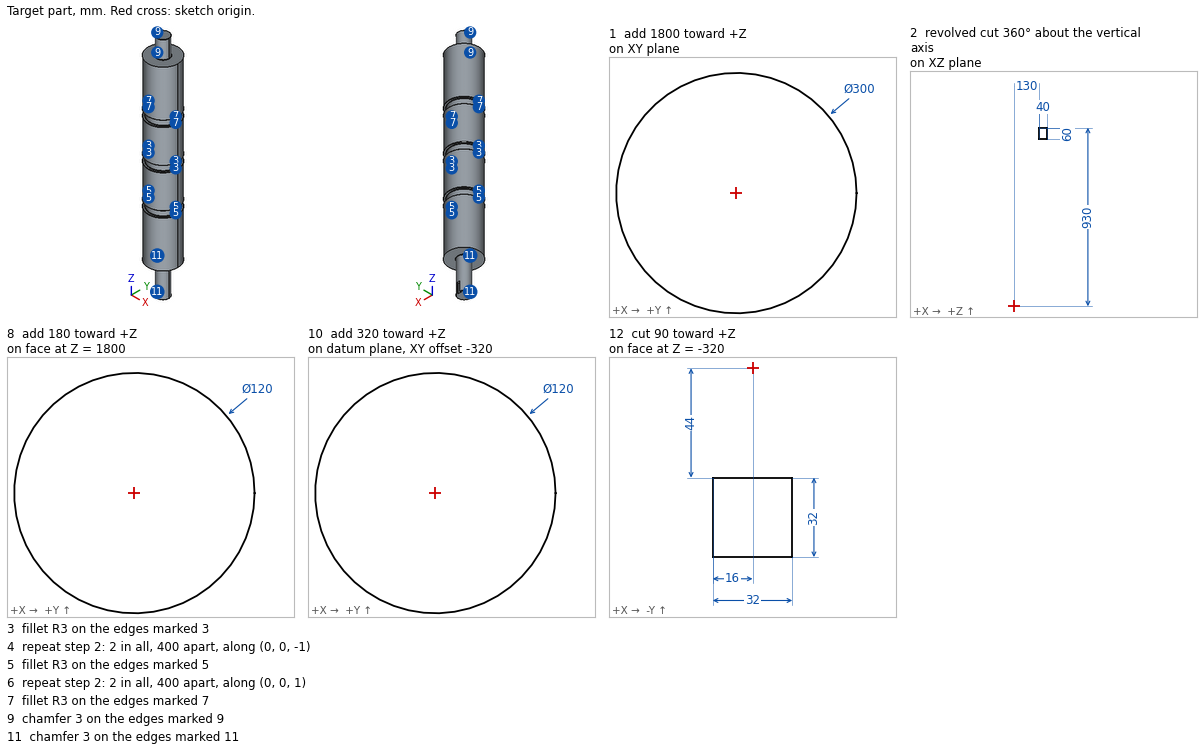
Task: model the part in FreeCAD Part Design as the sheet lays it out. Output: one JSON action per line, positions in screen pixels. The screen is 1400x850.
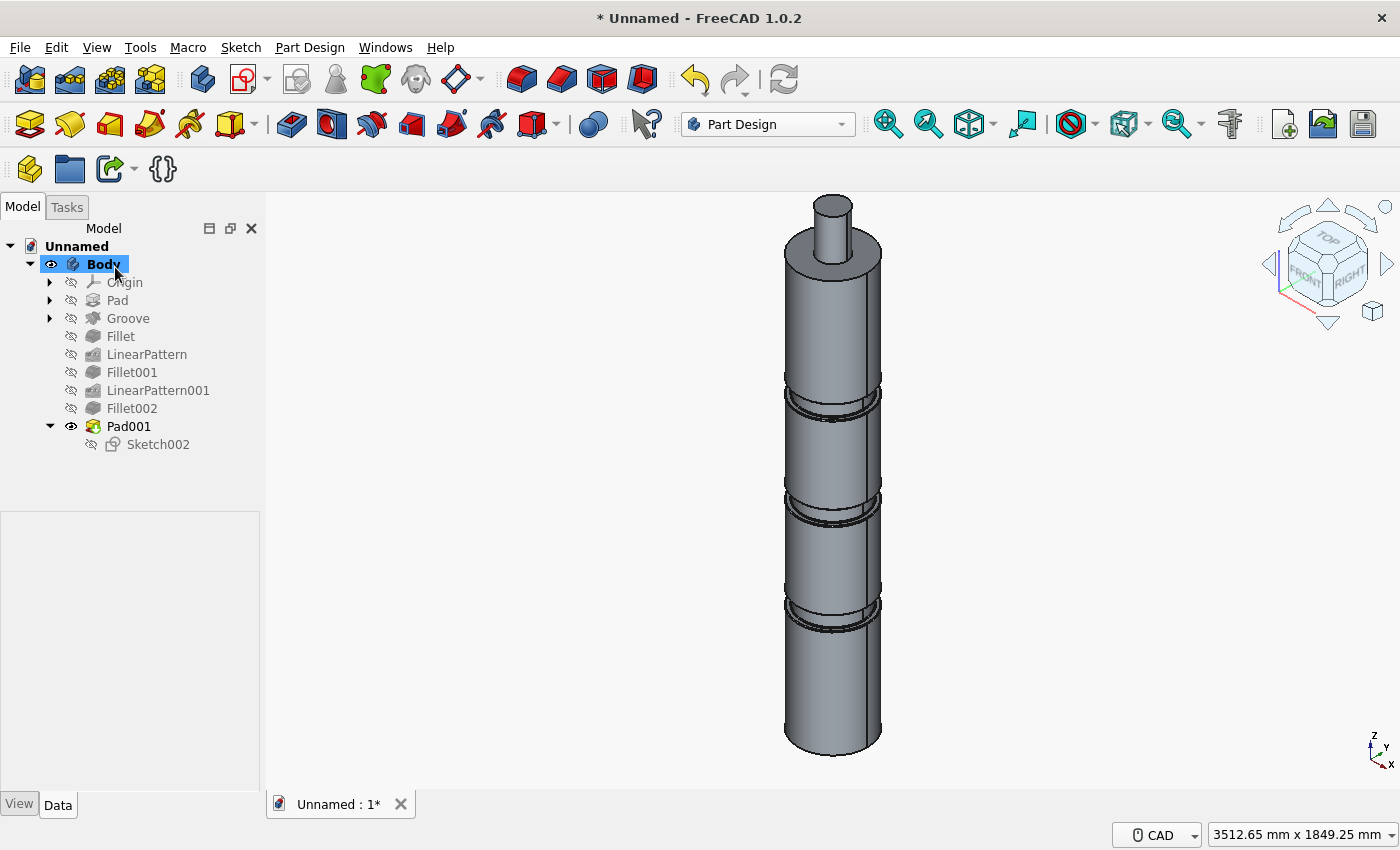
{"action": "left_click", "coordinate": [890, 124]}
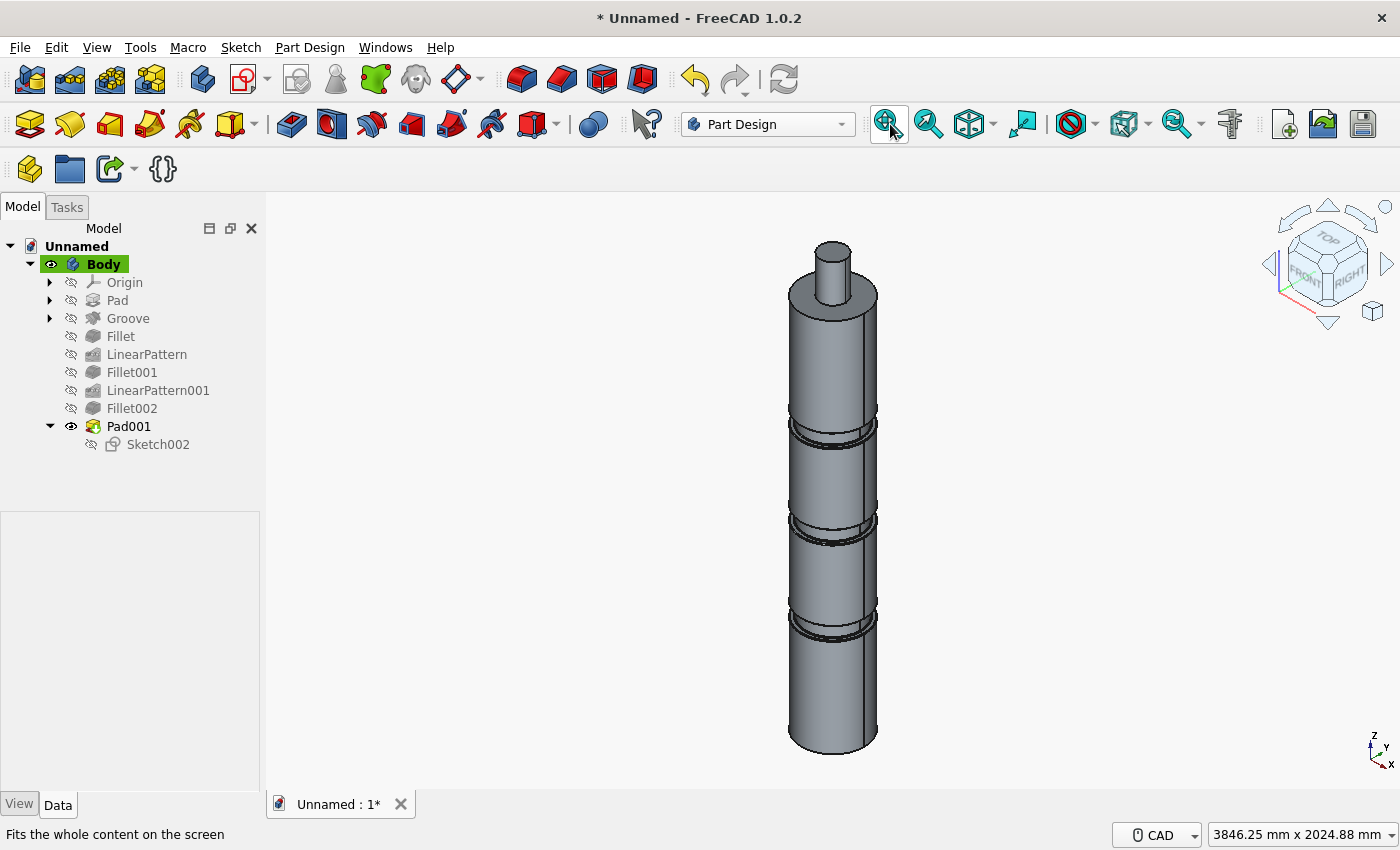
{"action": "left_click", "coordinate": [817, 299]}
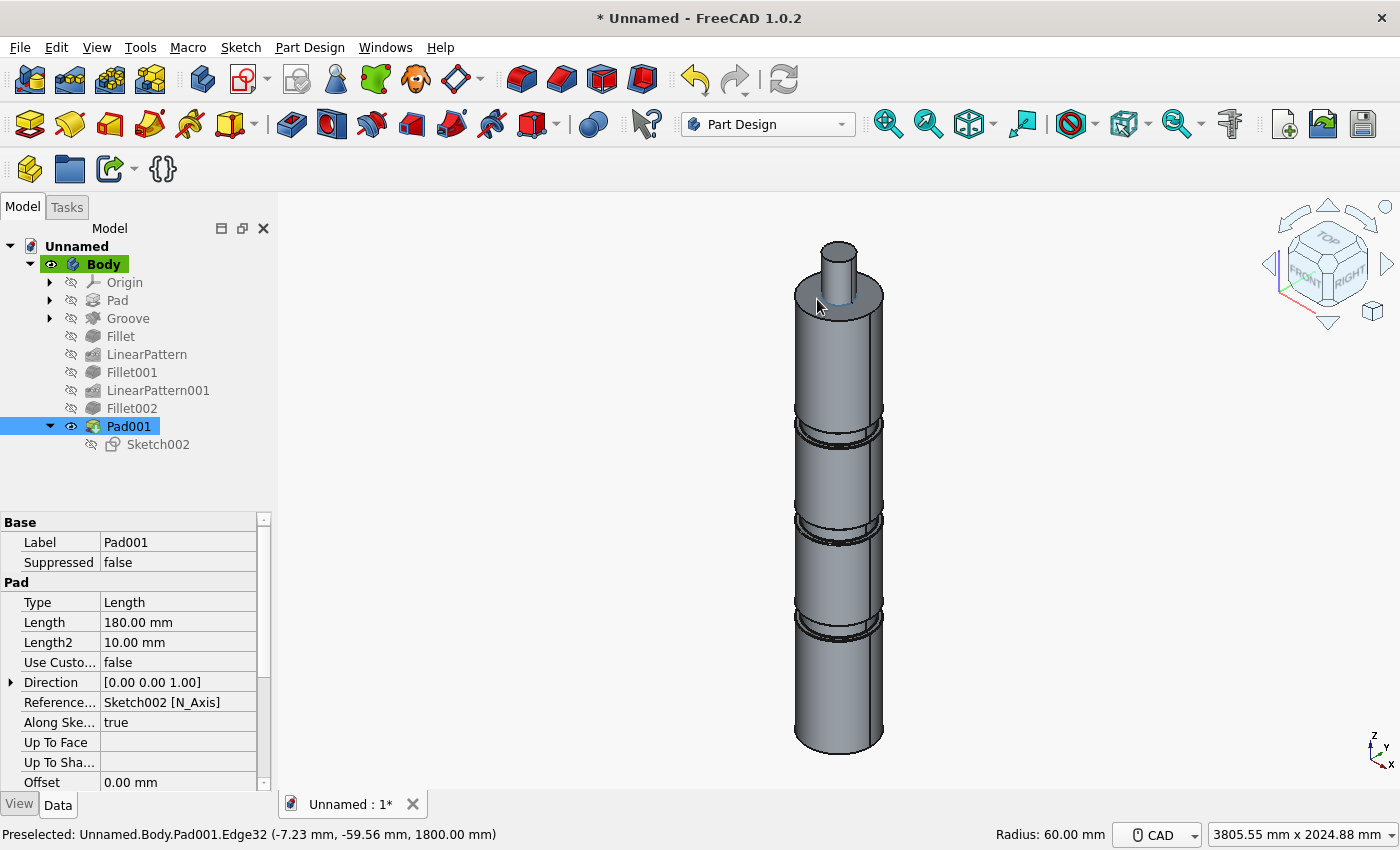
{"action": "left_click", "coordinate": [826, 244], "text": "ctrl"}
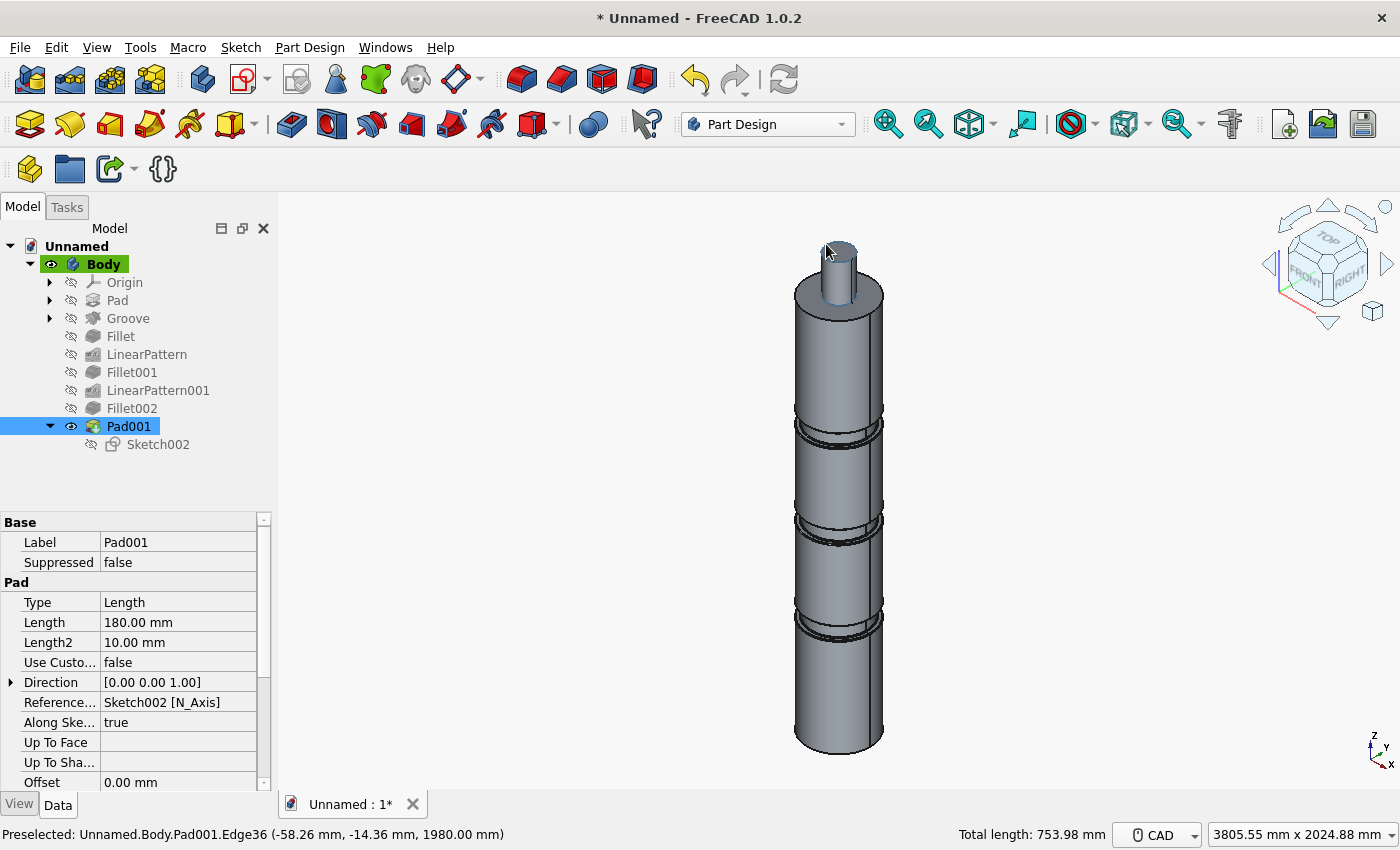
{"action": "left_click", "coordinate": [562, 80]}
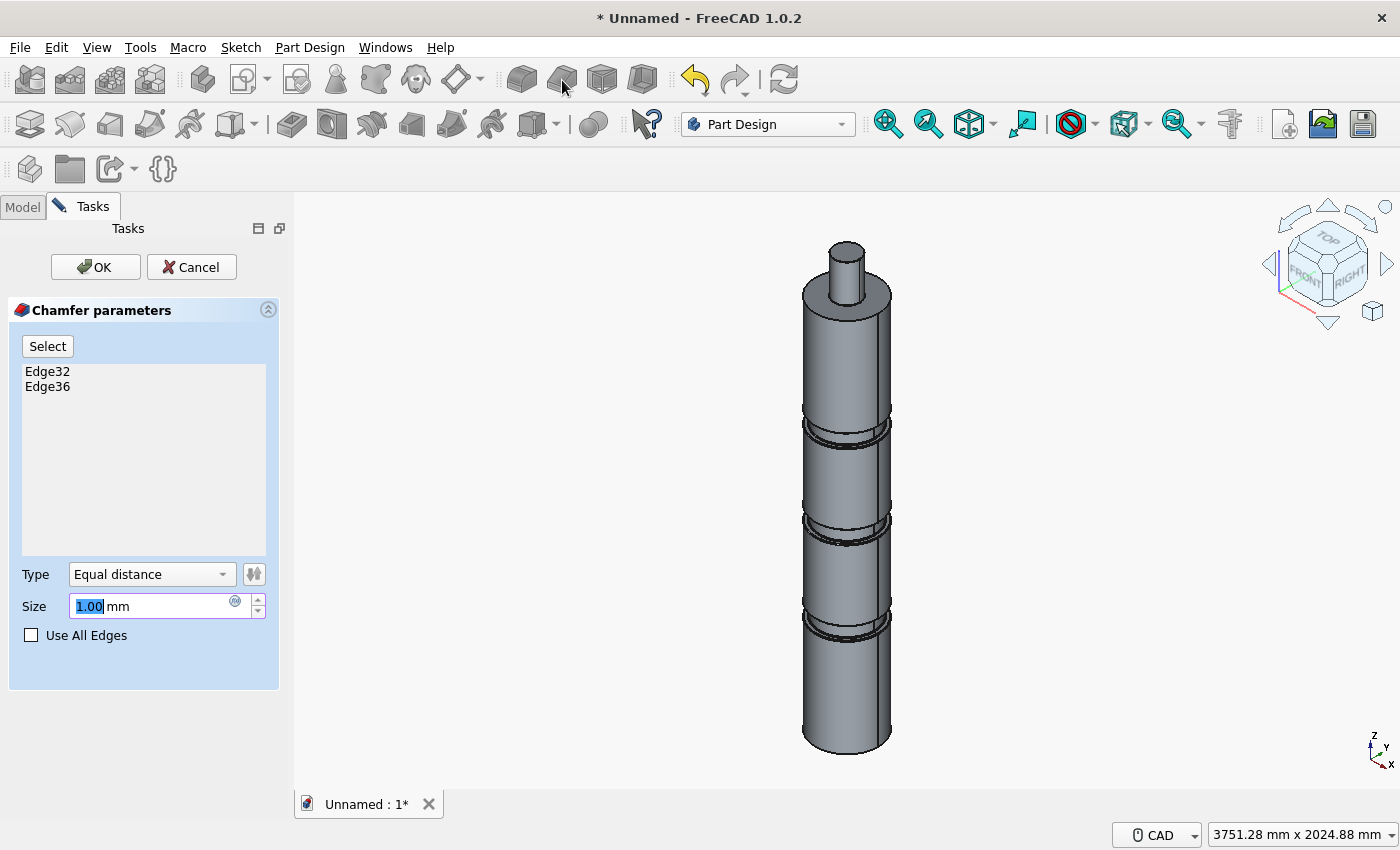
{"action": "type", "text": "3"}
{"action": "key", "text": "Tab"}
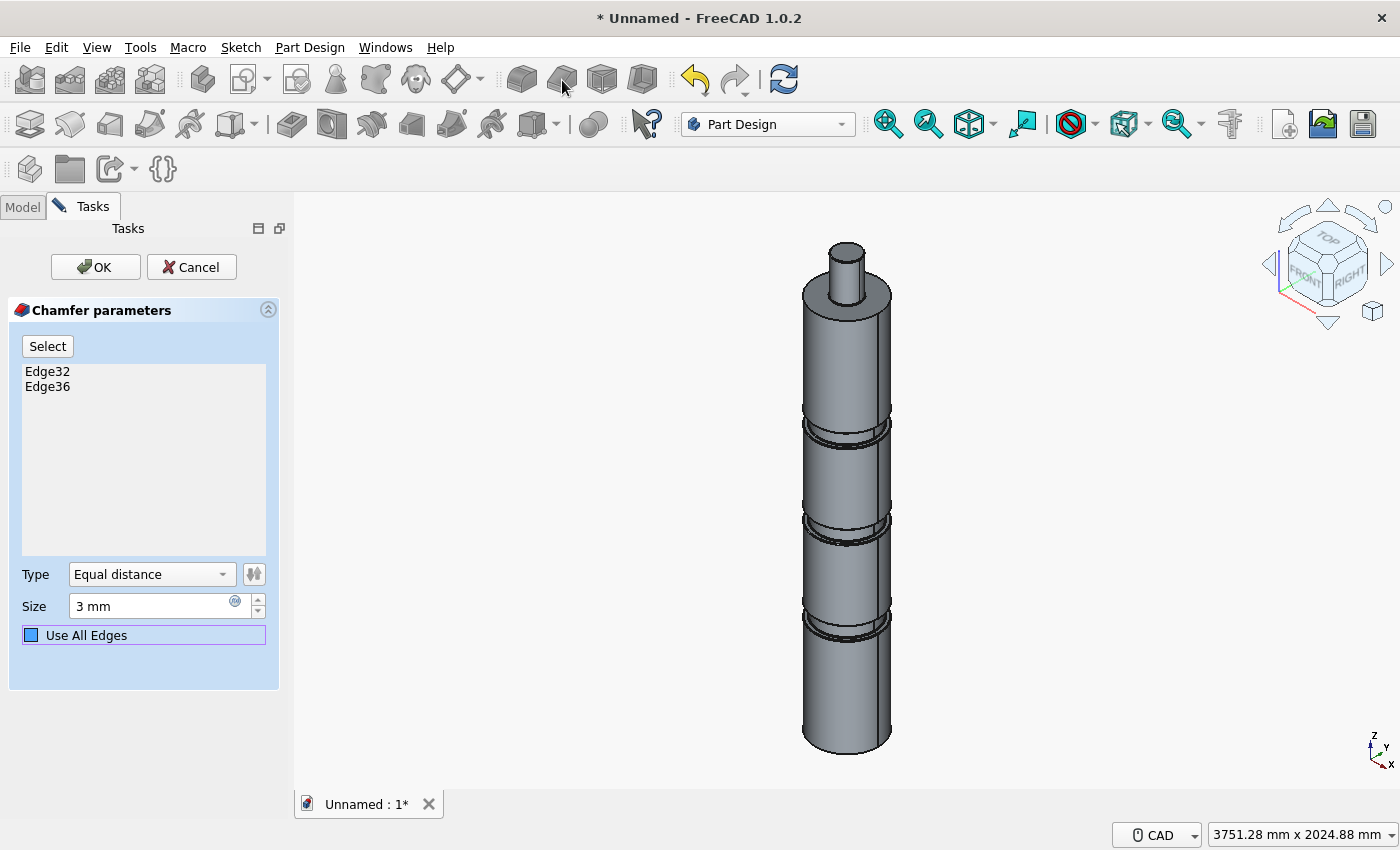
{"action": "left_click", "coordinate": [96, 267]}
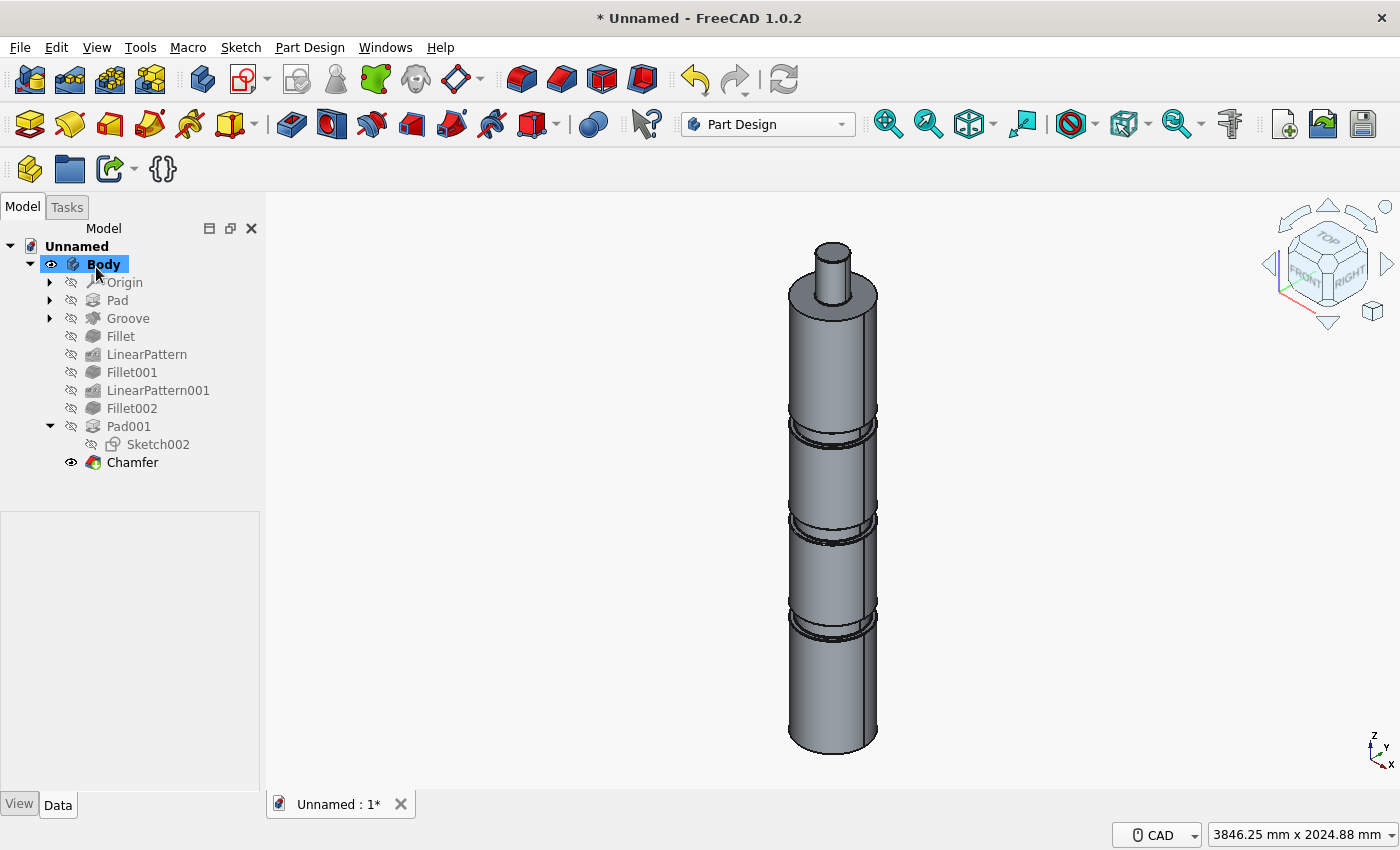
{"action": "left_click", "coordinate": [50, 282]}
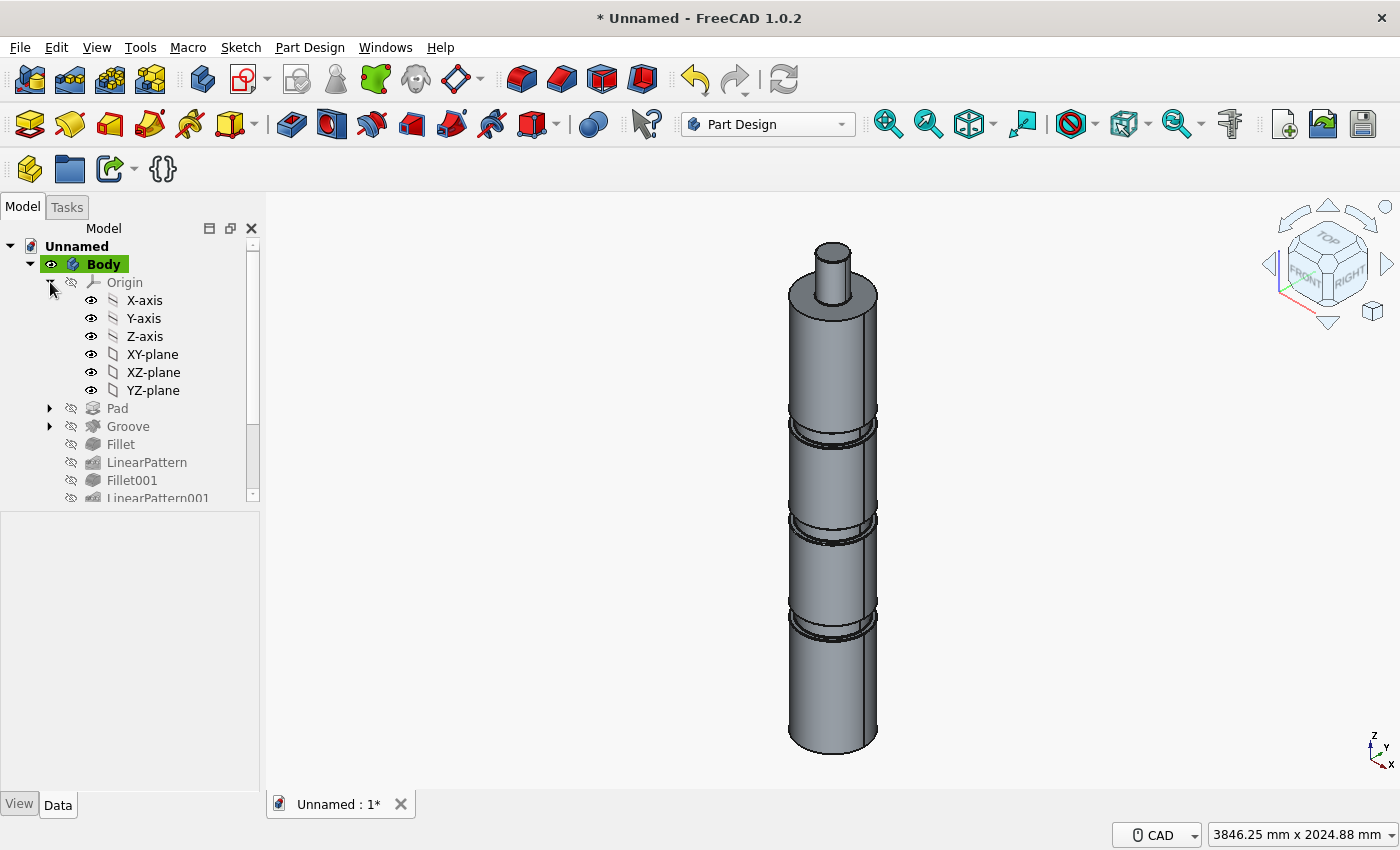
{"action": "left_click", "coordinate": [136, 354]}